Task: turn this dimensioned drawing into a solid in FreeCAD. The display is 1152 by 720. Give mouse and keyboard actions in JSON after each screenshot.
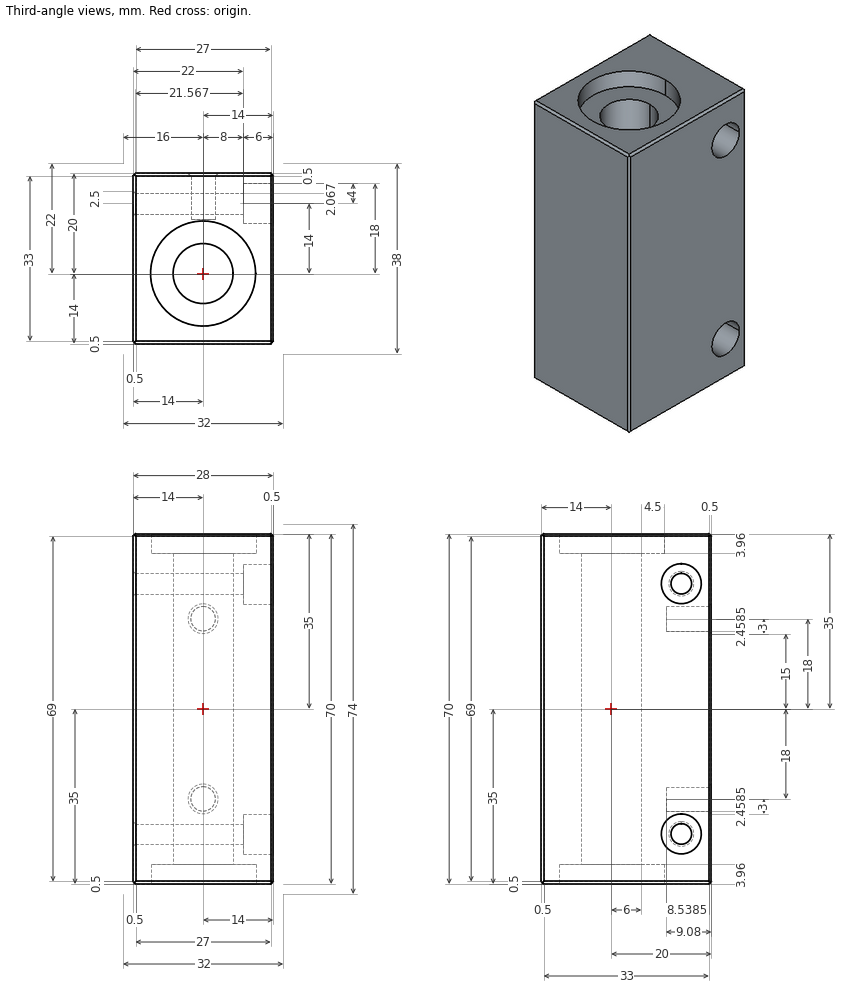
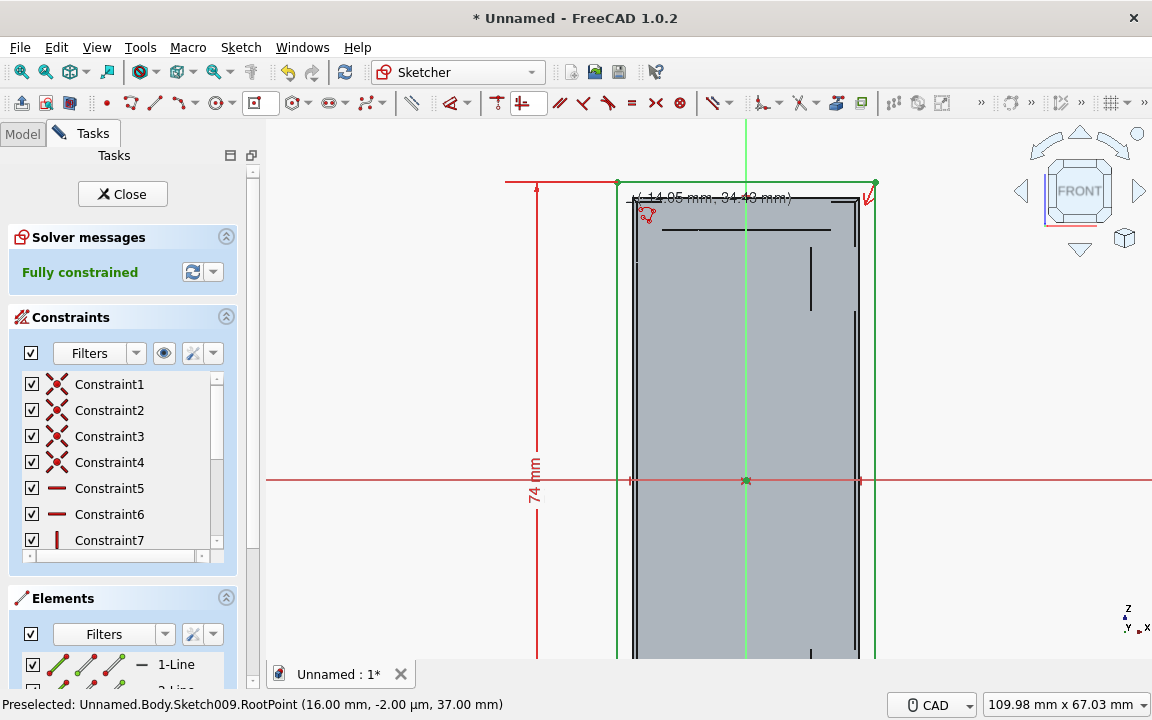
{"action": "scroll", "coordinate": [512, 278], "scroll_direction": "down", "scroll_amount": 3}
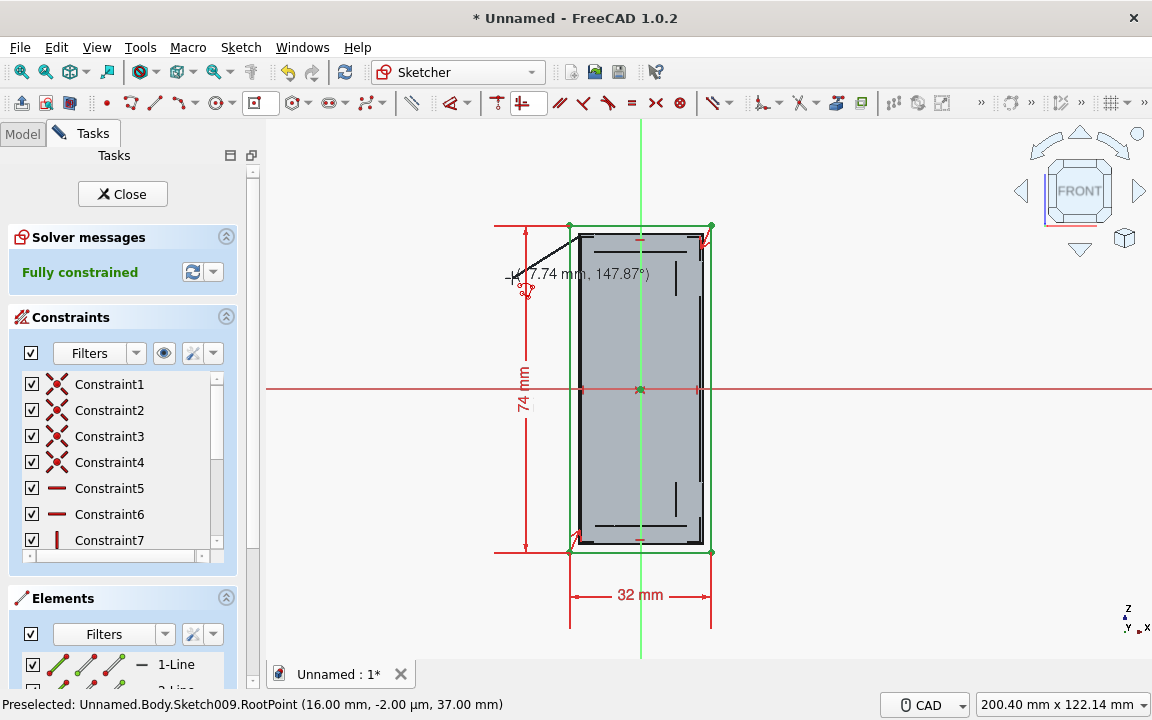
{"action": "scroll", "coordinate": [579, 542], "scroll_direction": "up", "scroll_amount": 3}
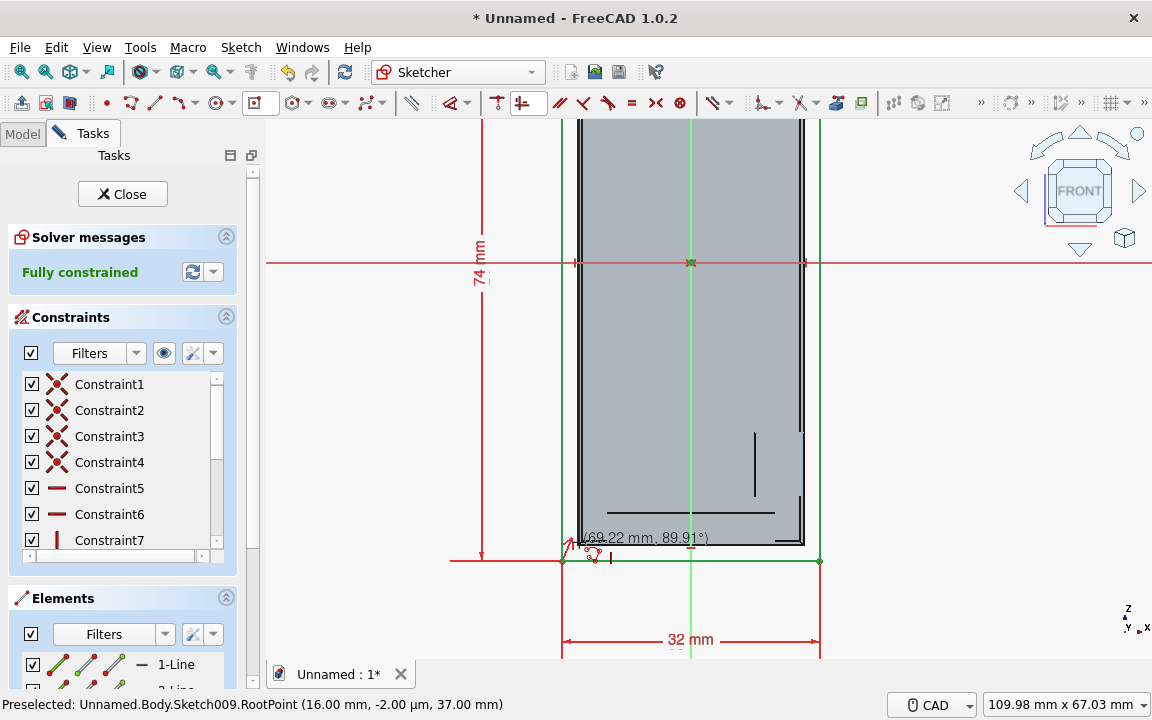
{"action": "left_click", "coordinate": [578, 541]}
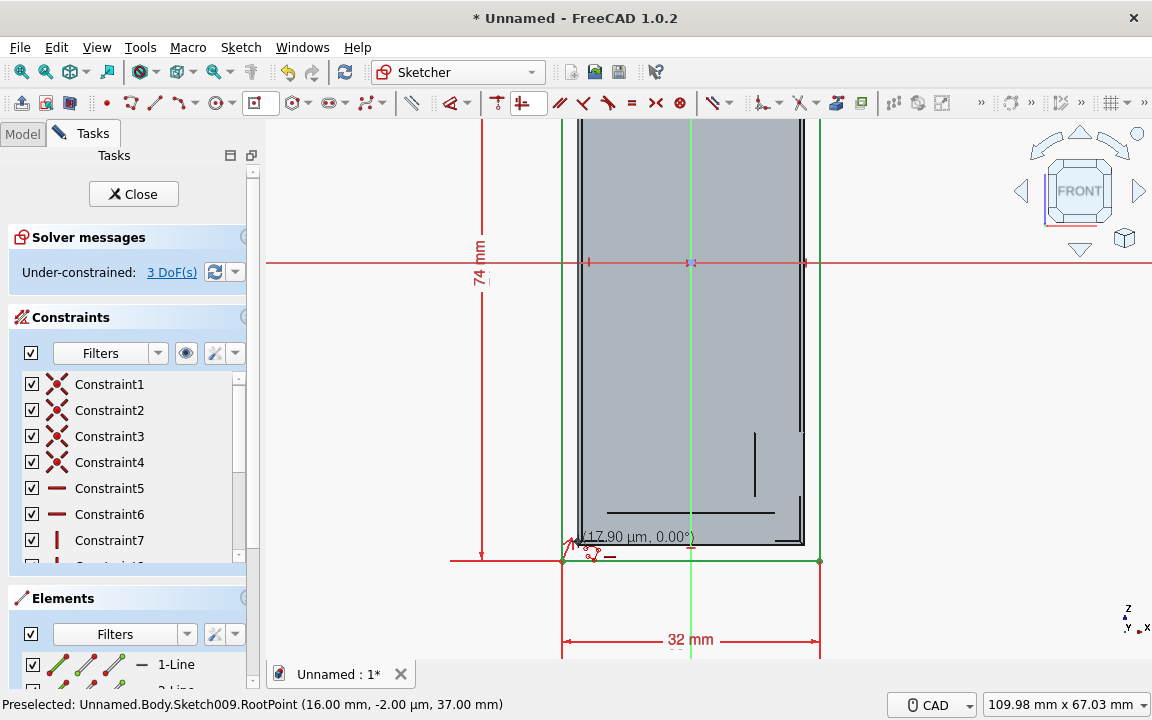
{"action": "scroll", "coordinate": [582, 545], "scroll_direction": "up", "scroll_amount": 6}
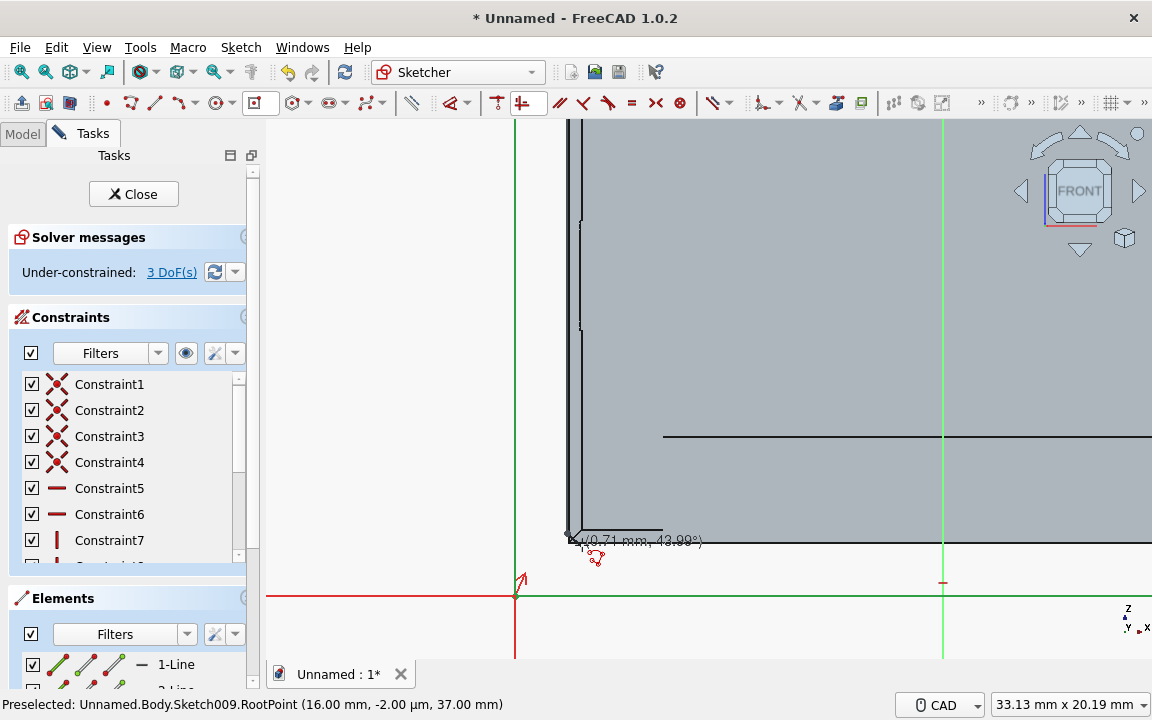
{"action": "left_click", "coordinate": [582, 543]}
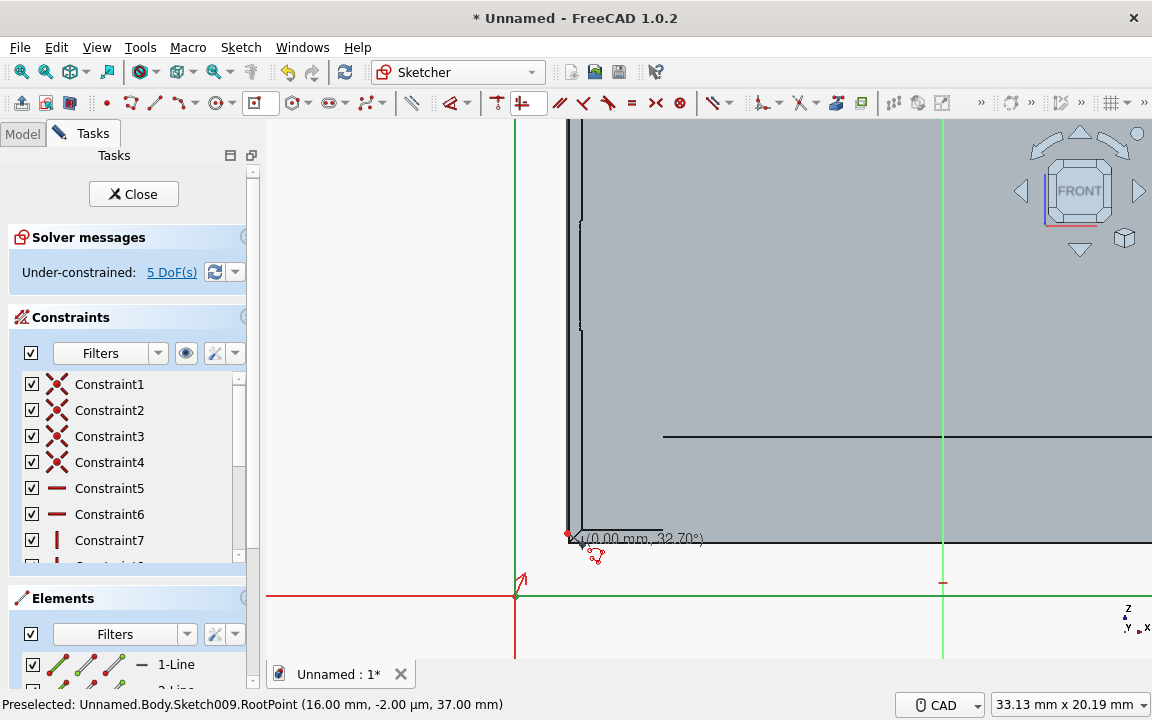
{"action": "scroll", "coordinate": [581, 544], "scroll_direction": "down", "scroll_amount": 9}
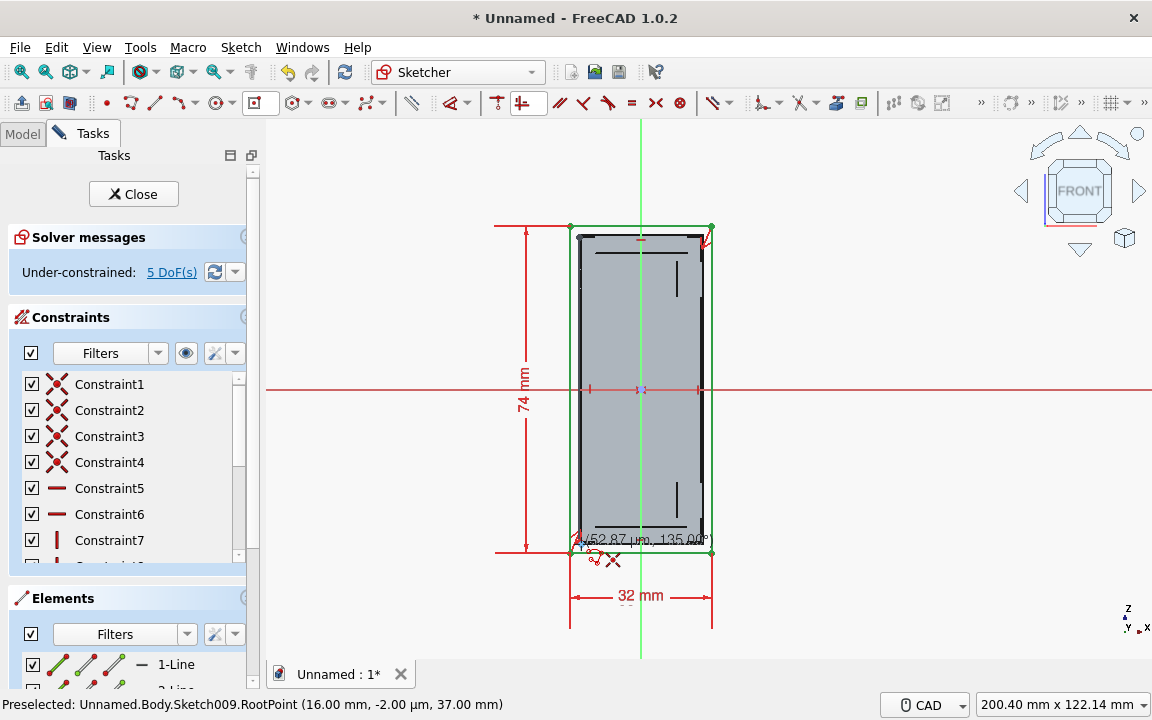
{"action": "scroll", "coordinate": [701, 544], "scroll_direction": "up", "scroll_amount": 3}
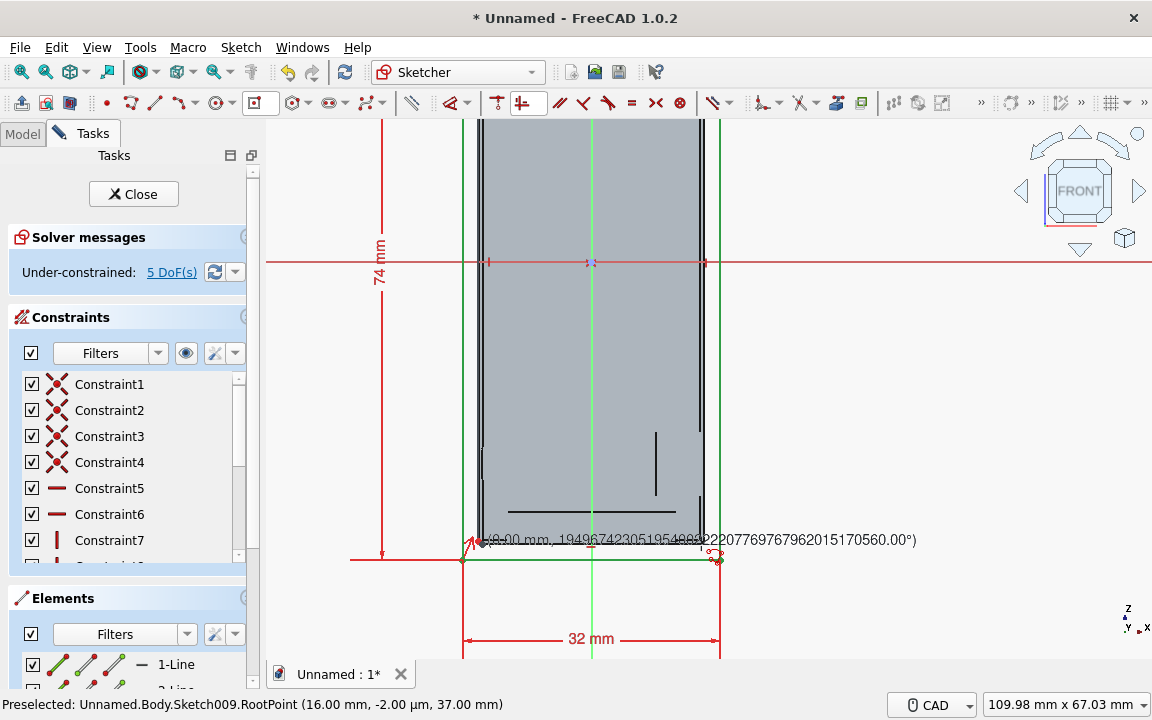
{"action": "left_click", "coordinate": [700, 544]}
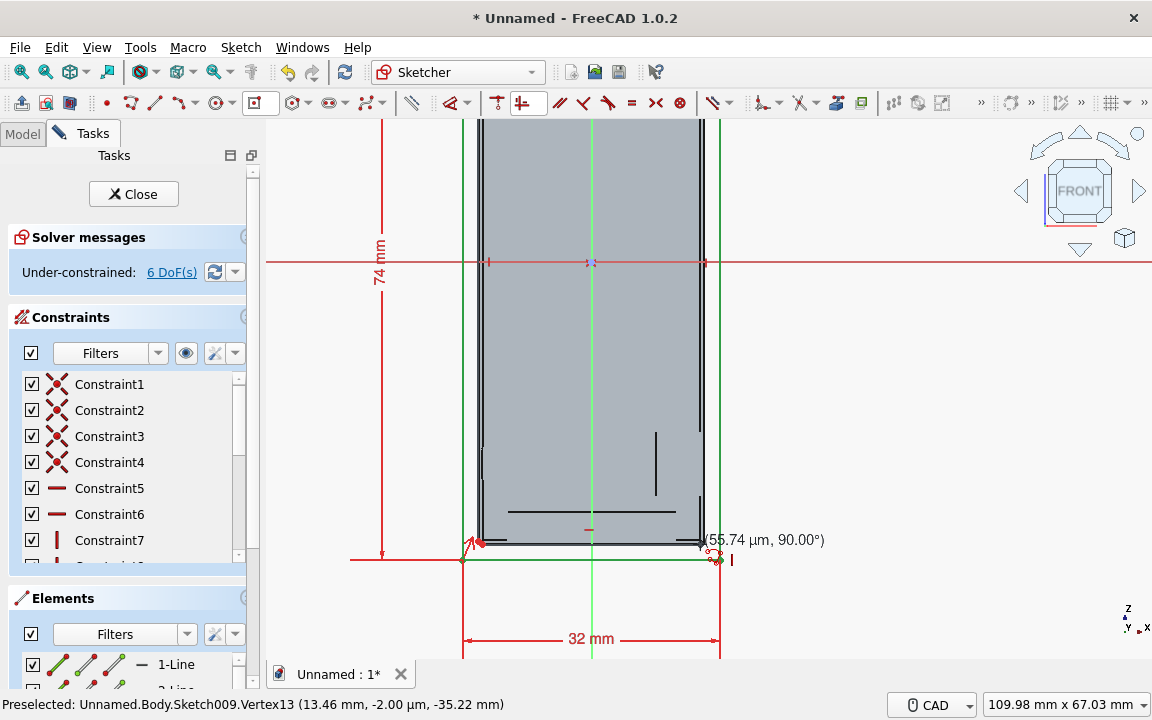
{"action": "scroll", "coordinate": [704, 540], "scroll_direction": "up", "scroll_amount": 6}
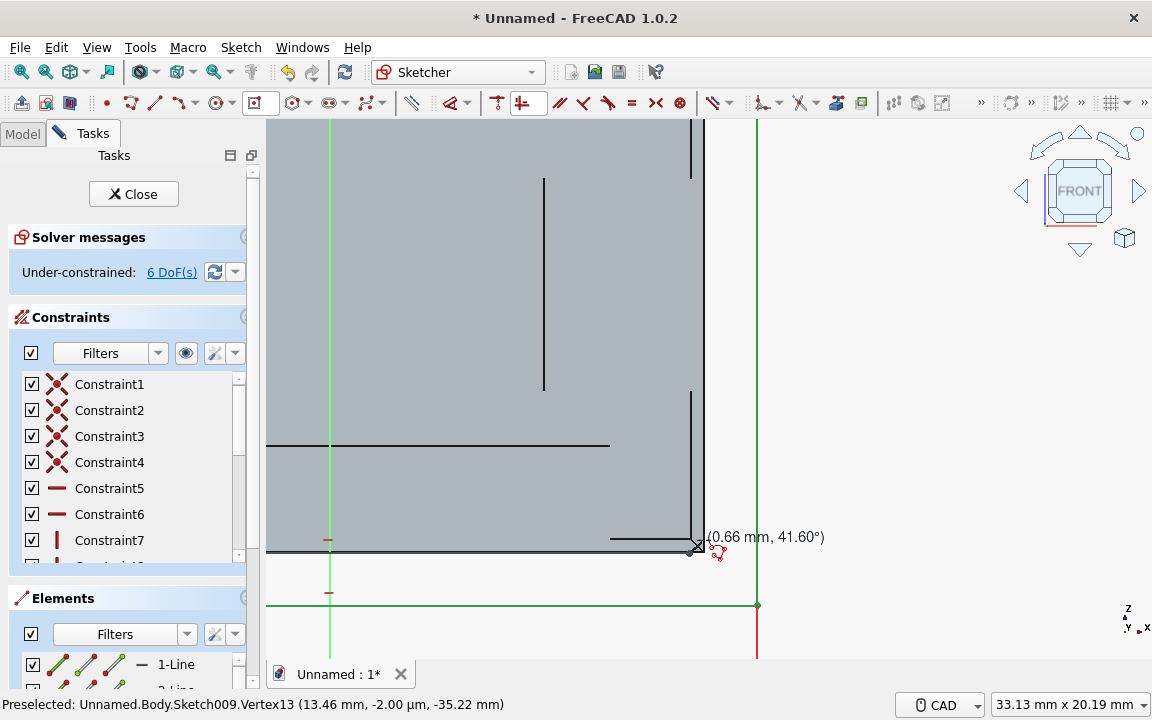
{"action": "left_click", "coordinate": [704, 539]}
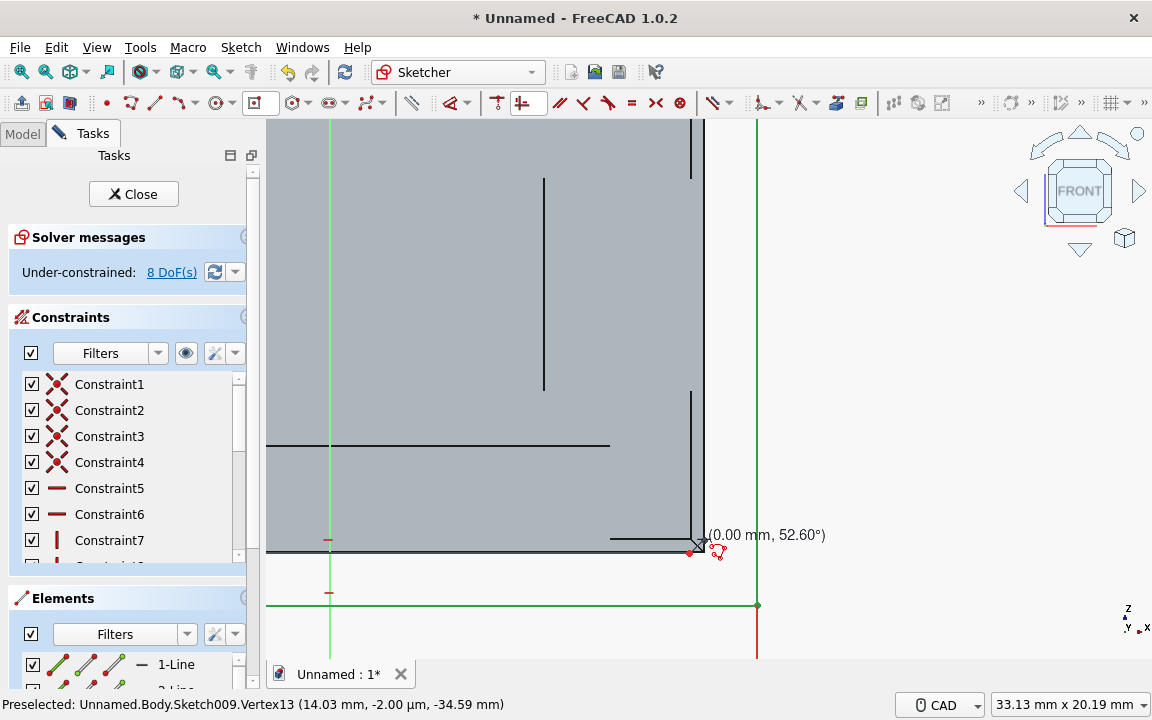
{"action": "scroll", "coordinate": [702, 542], "scroll_direction": "down", "scroll_amount": 9}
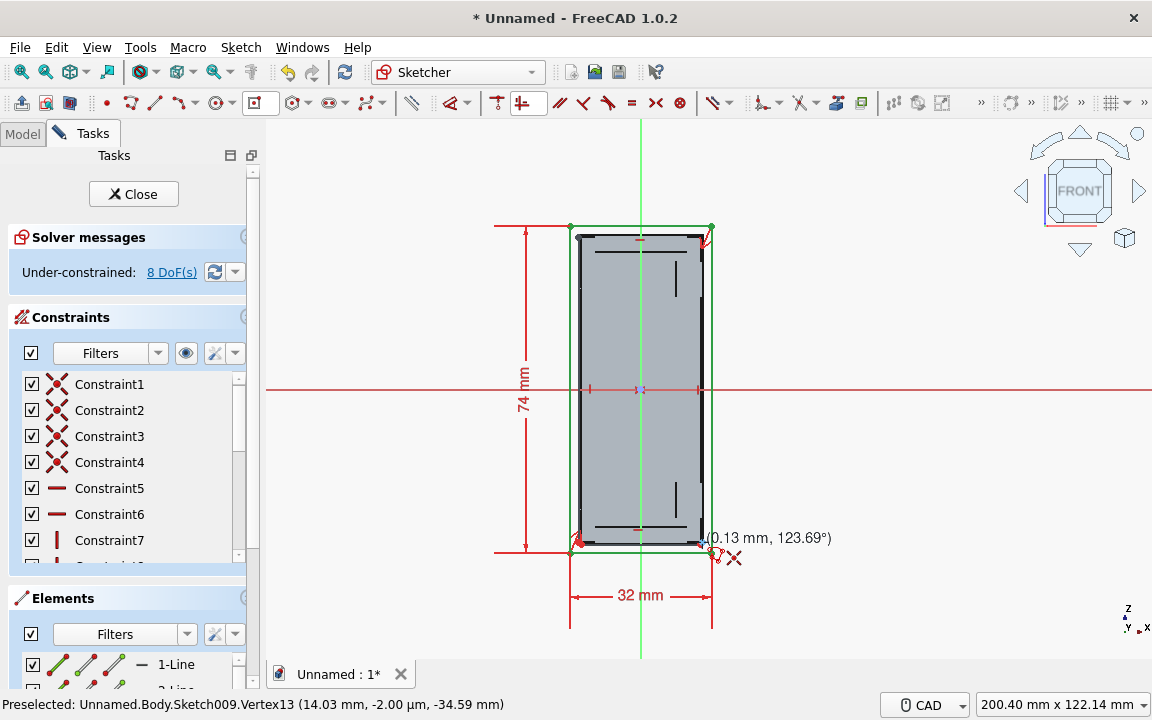
{"action": "scroll", "coordinate": [703, 237], "scroll_direction": "up", "scroll_amount": 3}